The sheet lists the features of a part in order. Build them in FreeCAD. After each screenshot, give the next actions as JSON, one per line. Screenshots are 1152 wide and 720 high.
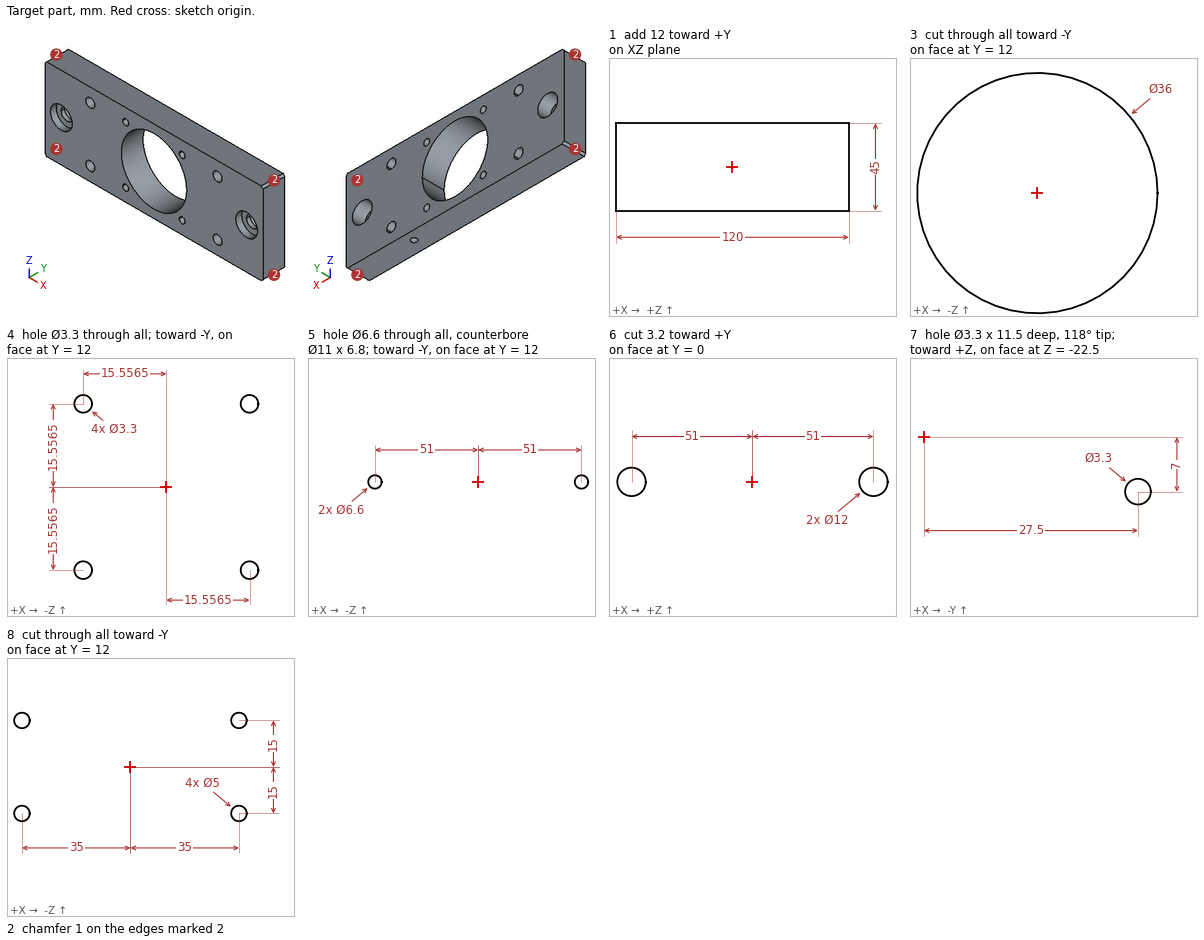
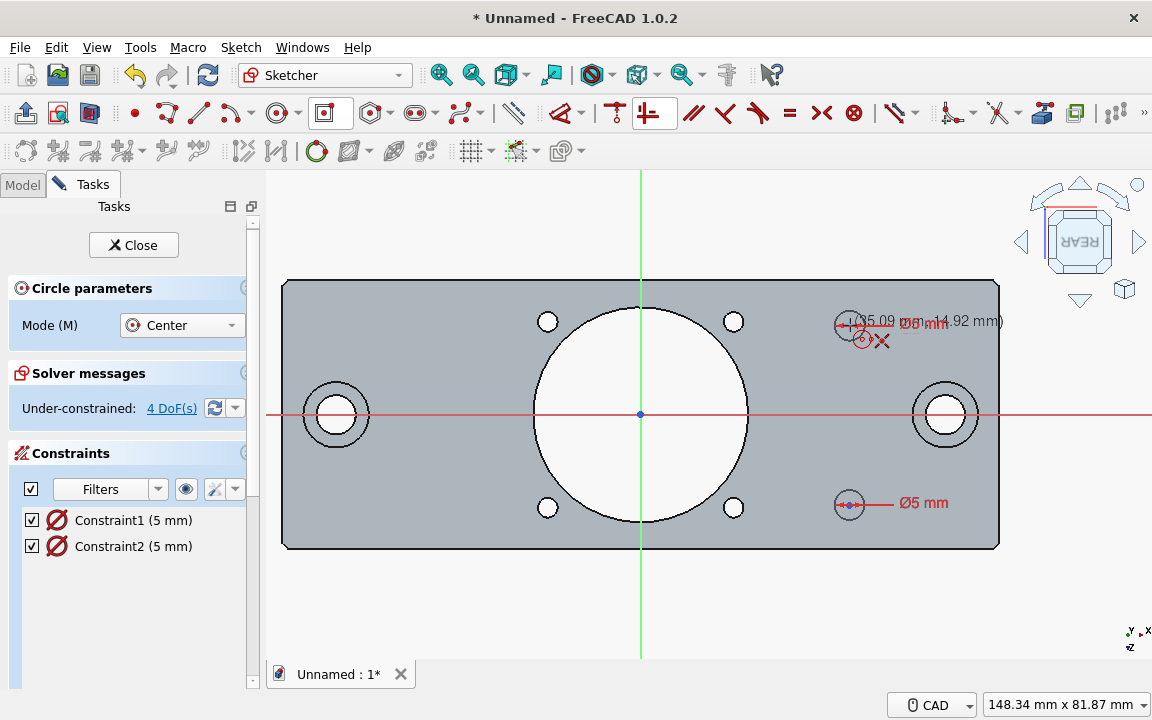
{"action": "scroll", "coordinate": [432, 504], "scroll_direction": "up", "scroll_amount": 3}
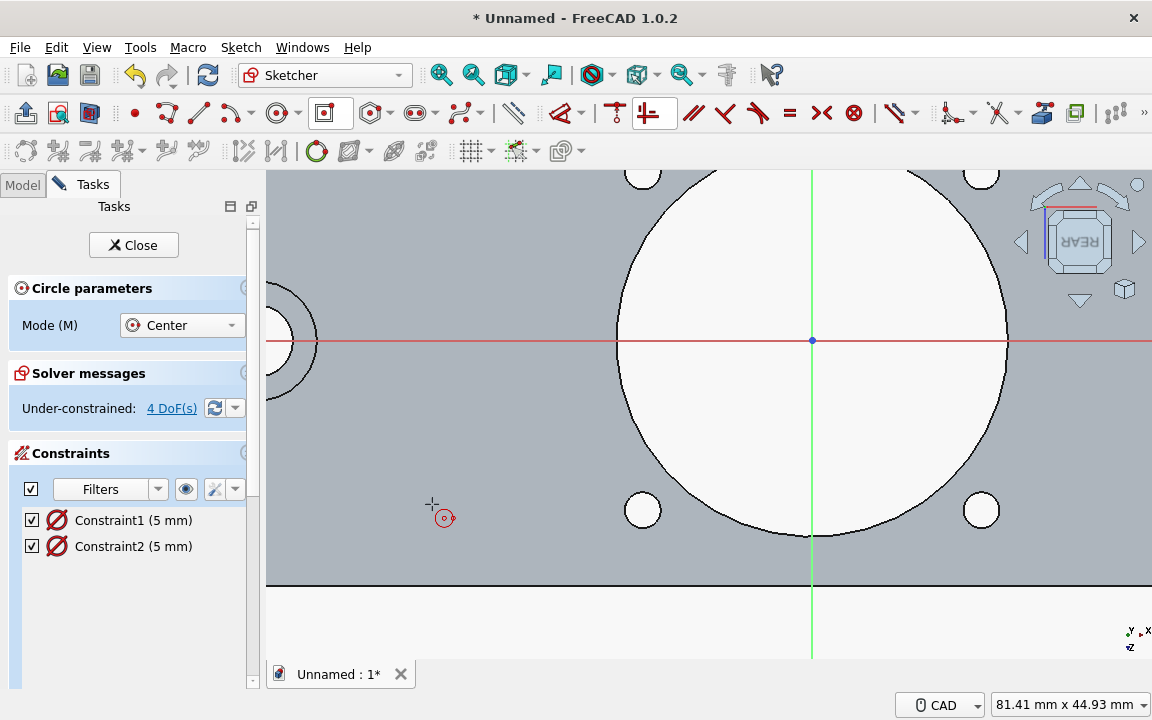
{"action": "left_click", "coordinate": [431, 504]}
{"action": "mouse_move", "coordinate": [451, 485]}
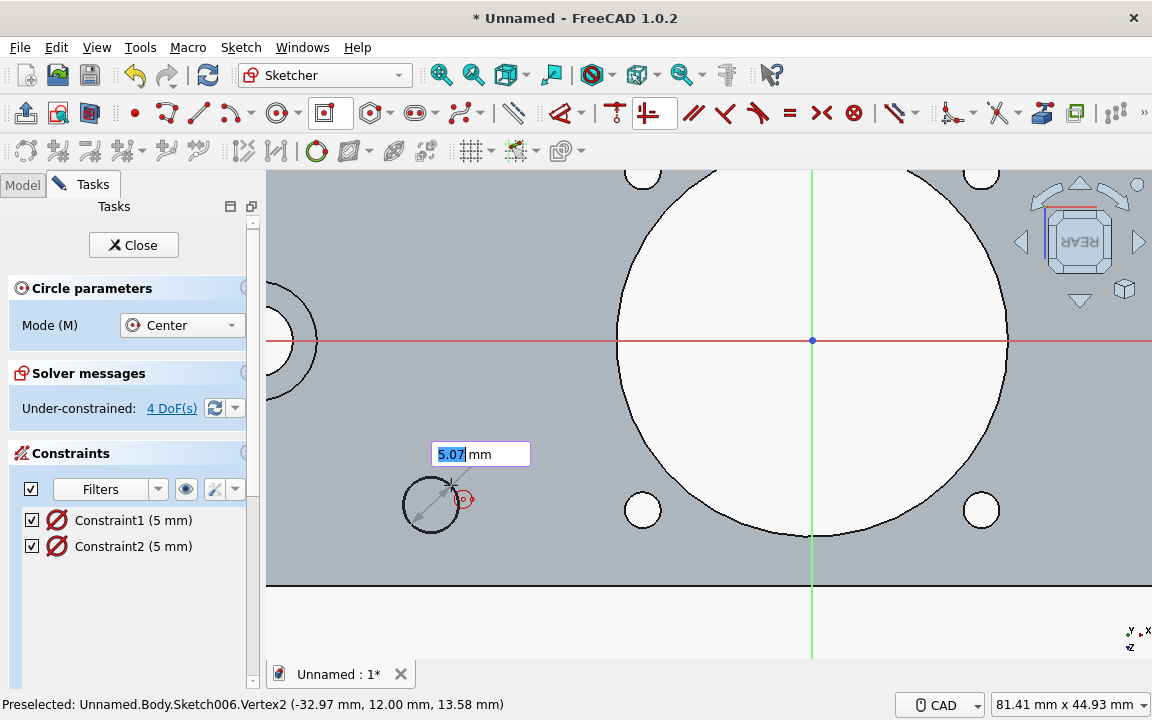
{"action": "type", "text": "5"}
{"action": "key", "text": "Return"}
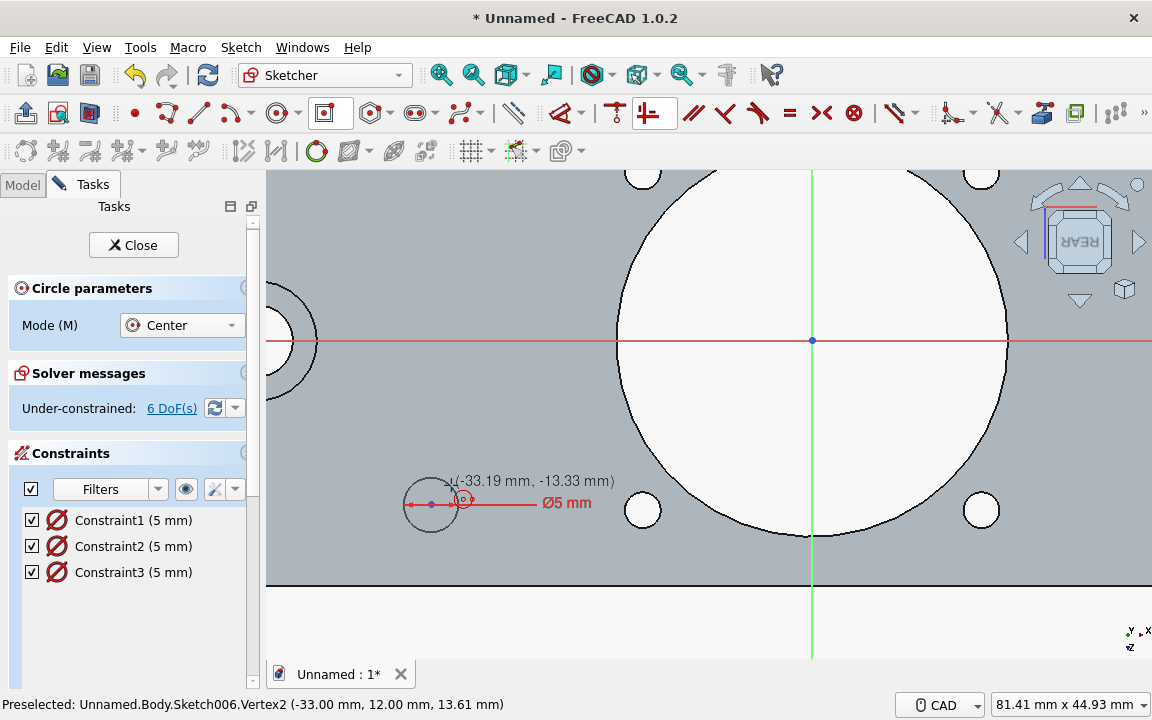
{"action": "scroll", "coordinate": [432, 504], "scroll_direction": "down", "scroll_amount": 3}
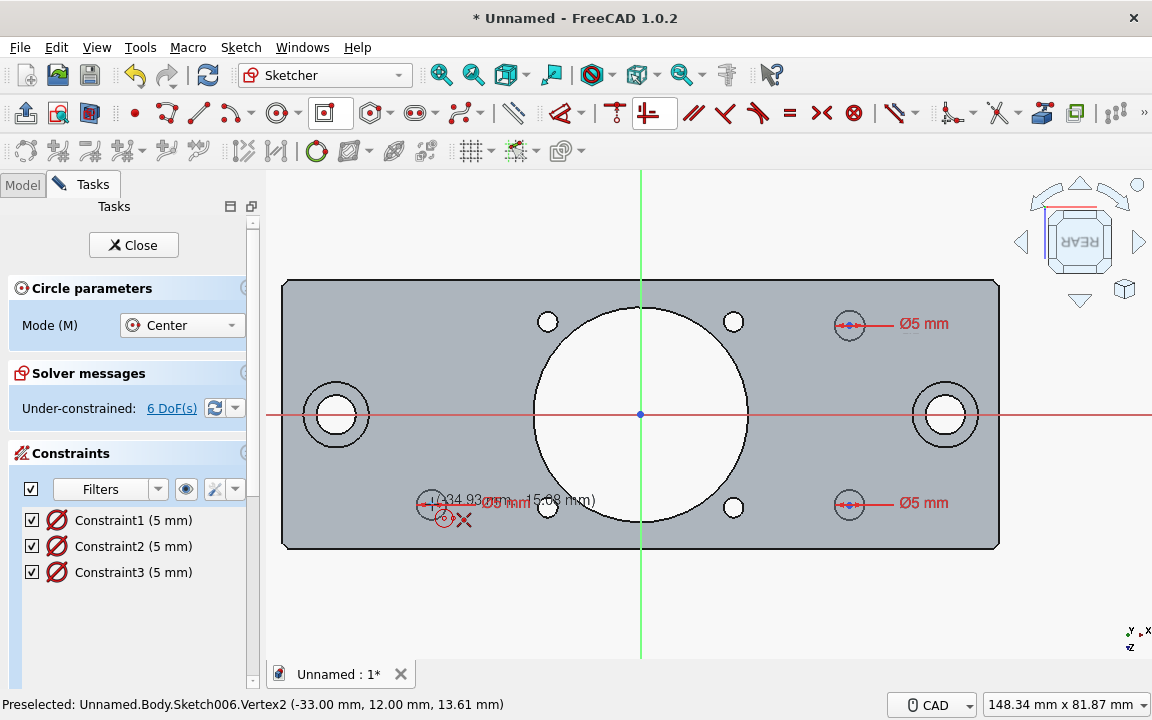
{"action": "scroll", "coordinate": [432, 325], "scroll_direction": "up", "scroll_amount": 3}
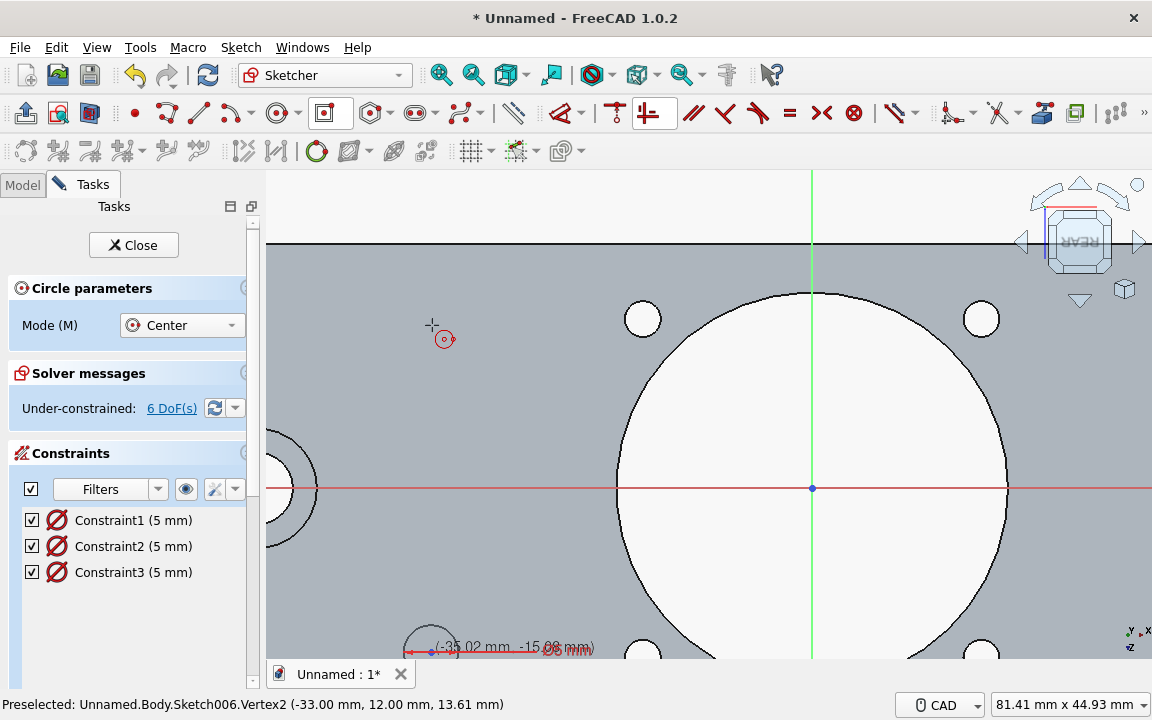
{"action": "left_click", "coordinate": [431, 325]}
{"action": "mouse_move", "coordinate": [451, 306]}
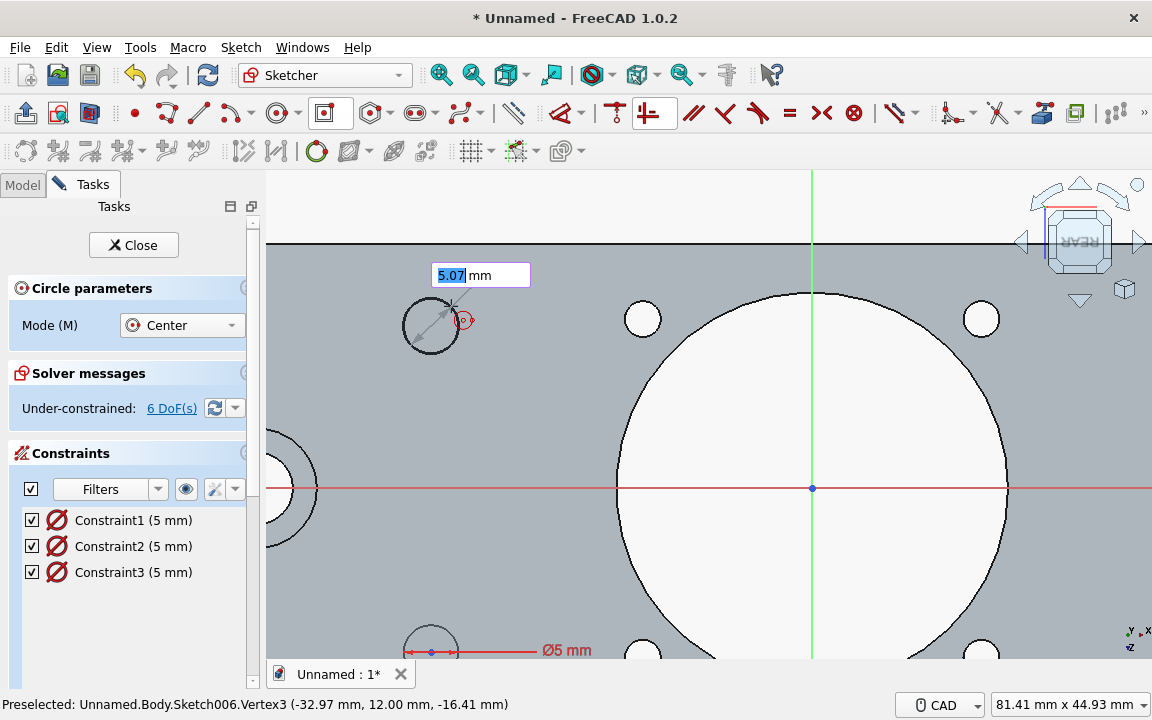
{"action": "type", "text": "5"}
{"action": "key", "text": "Return"}
{"action": "key", "text": "Escape"}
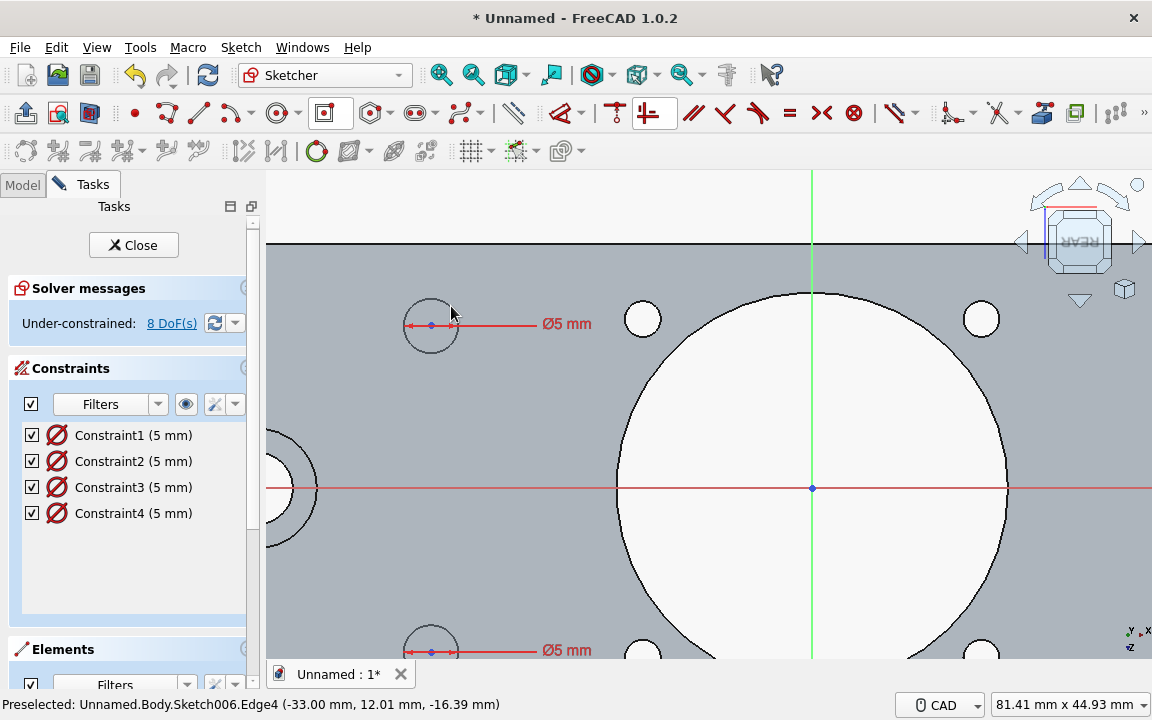
{"action": "scroll", "coordinate": [432, 325], "scroll_direction": "down", "scroll_amount": 3}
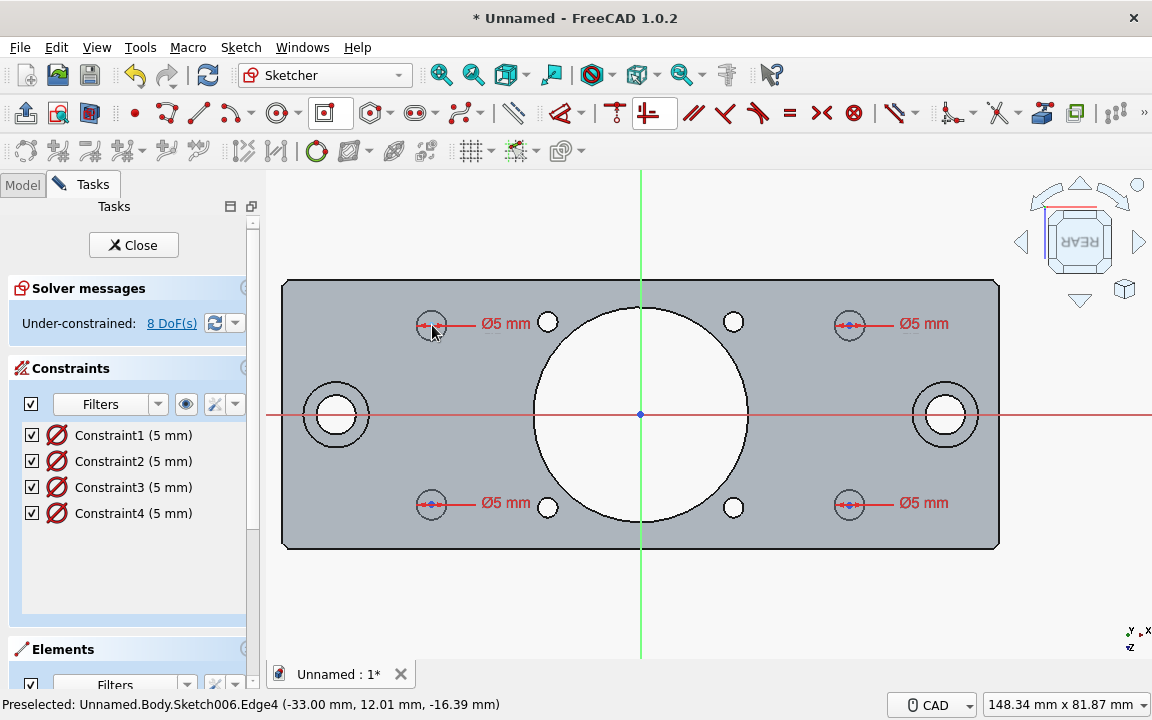
{"action": "left_click", "coordinate": [850, 505]}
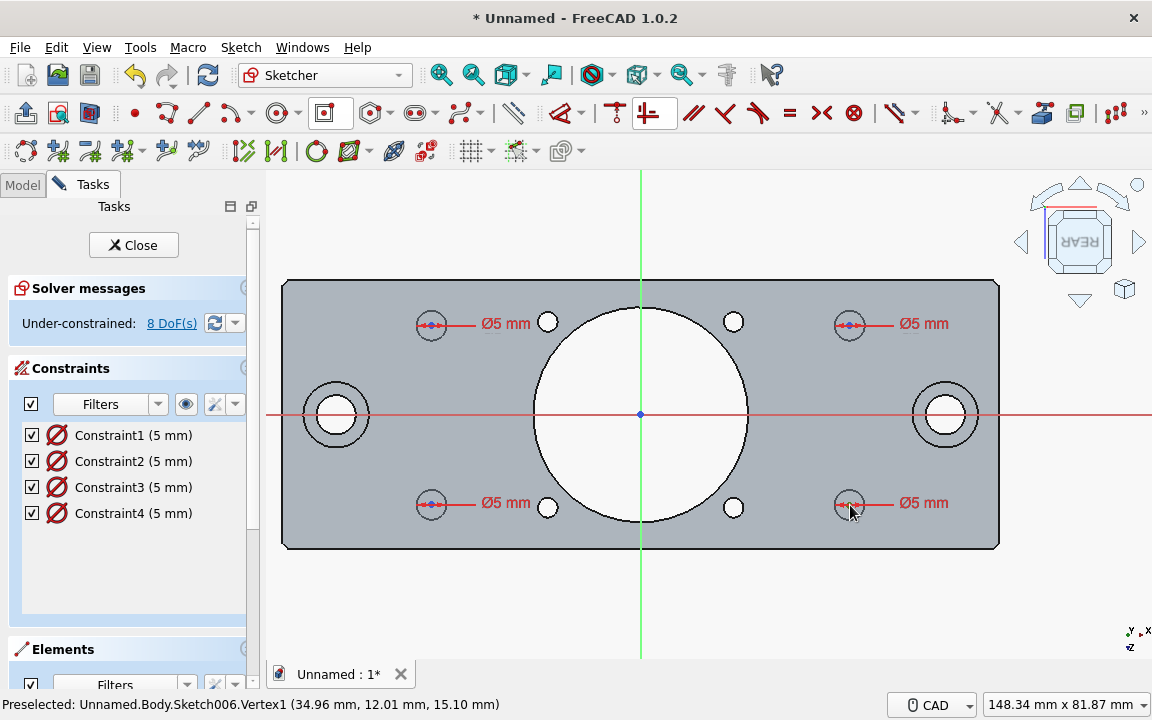
{"action": "left_click", "coordinate": [850, 326]}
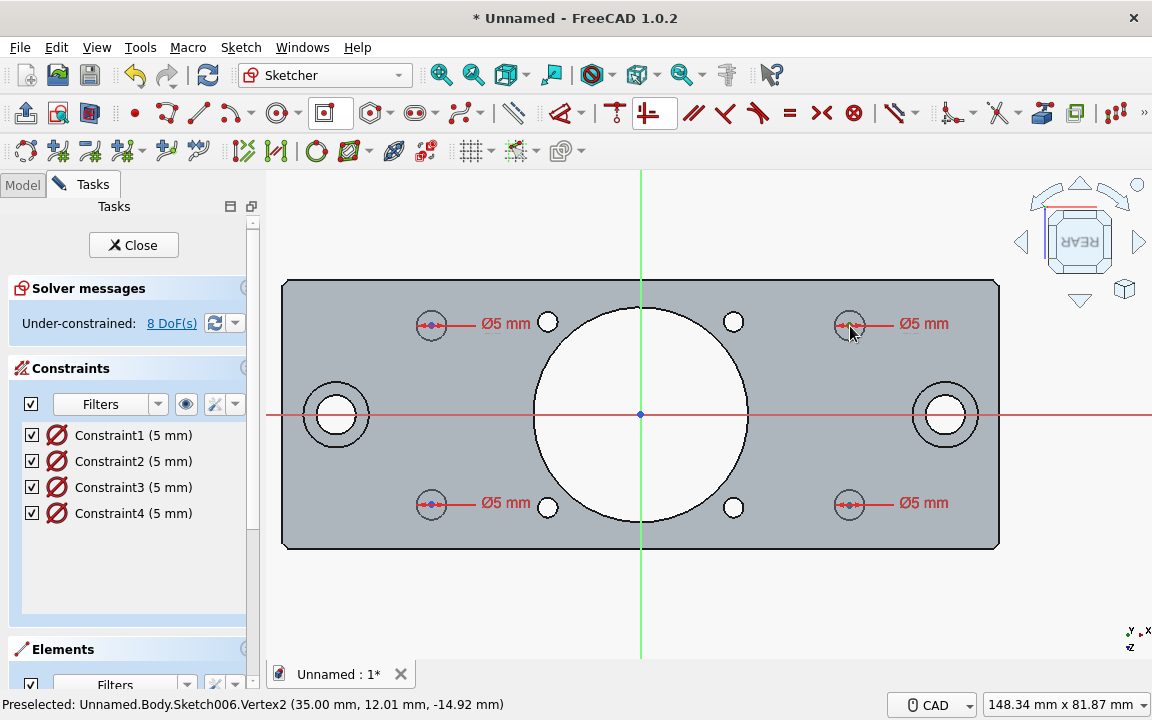
{"action": "key", "text": "v"}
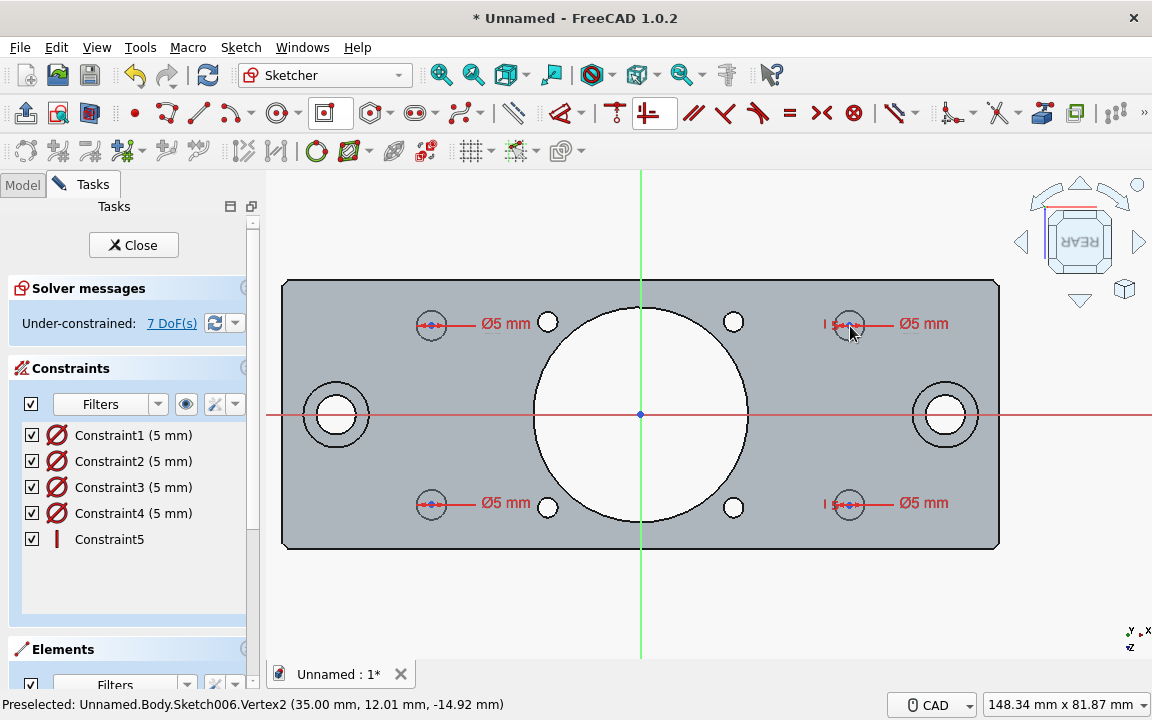
{"action": "left_click", "coordinate": [850, 505]}